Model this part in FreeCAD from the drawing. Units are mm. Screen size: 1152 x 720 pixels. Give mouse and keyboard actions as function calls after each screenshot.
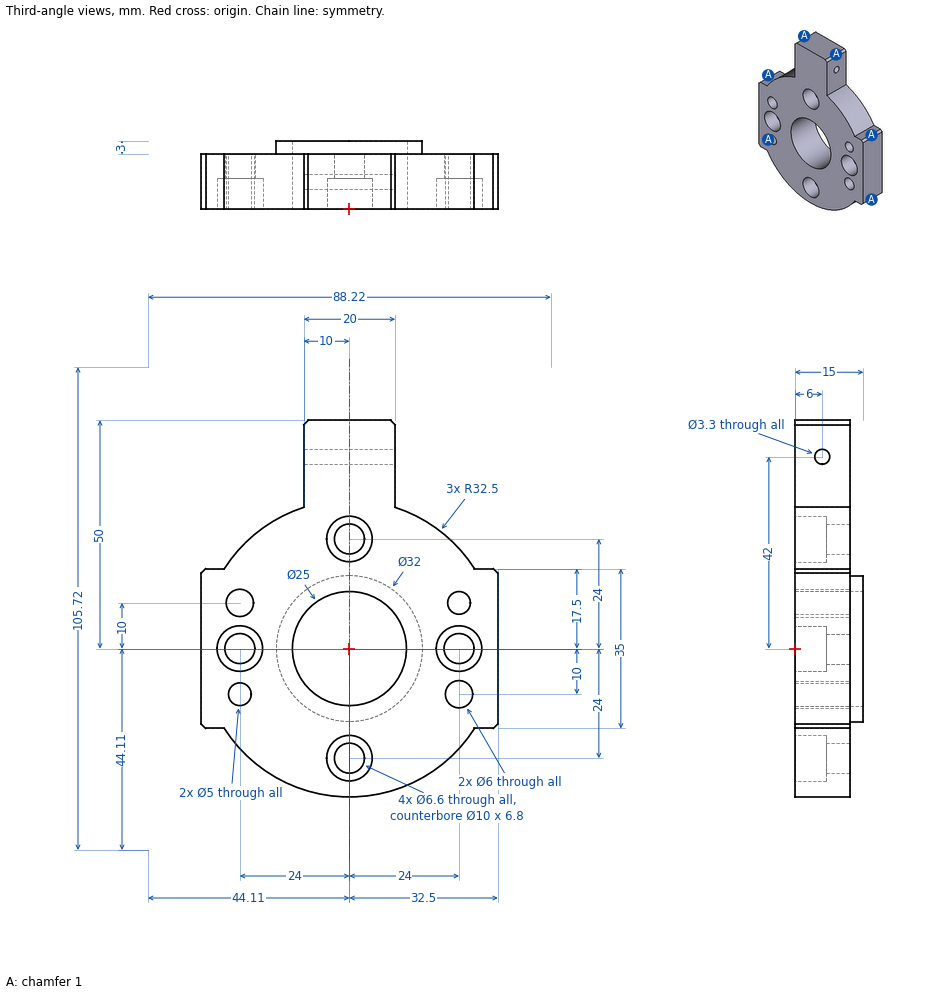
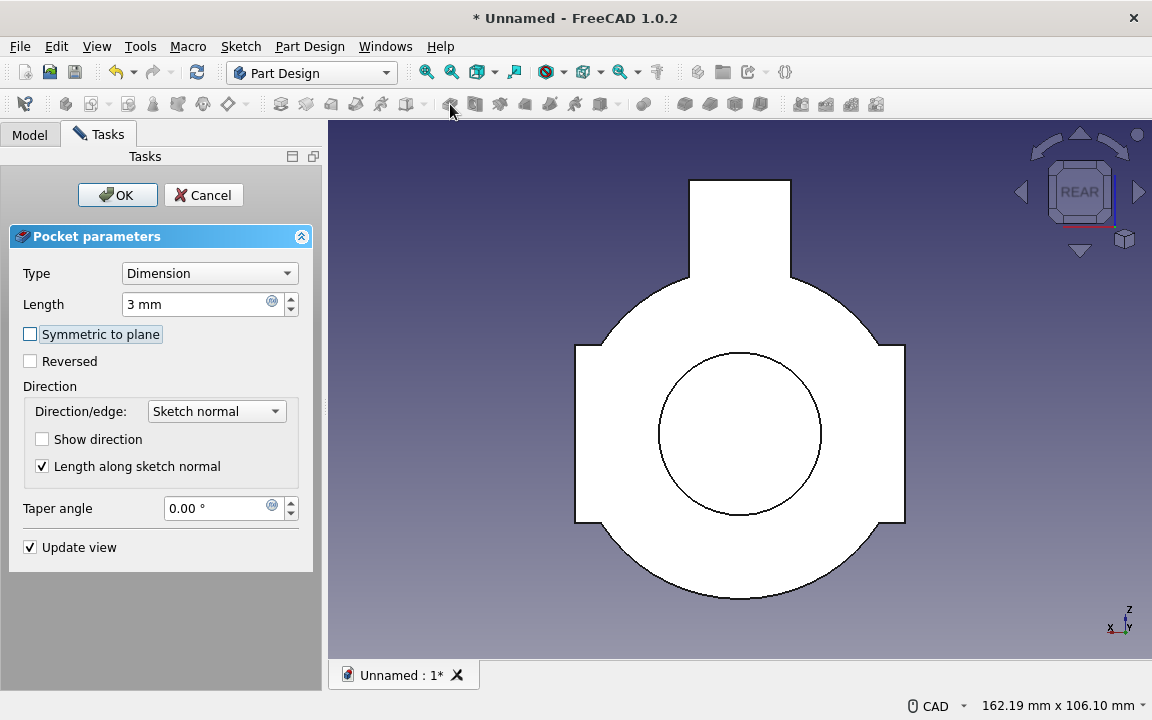
click(118, 195)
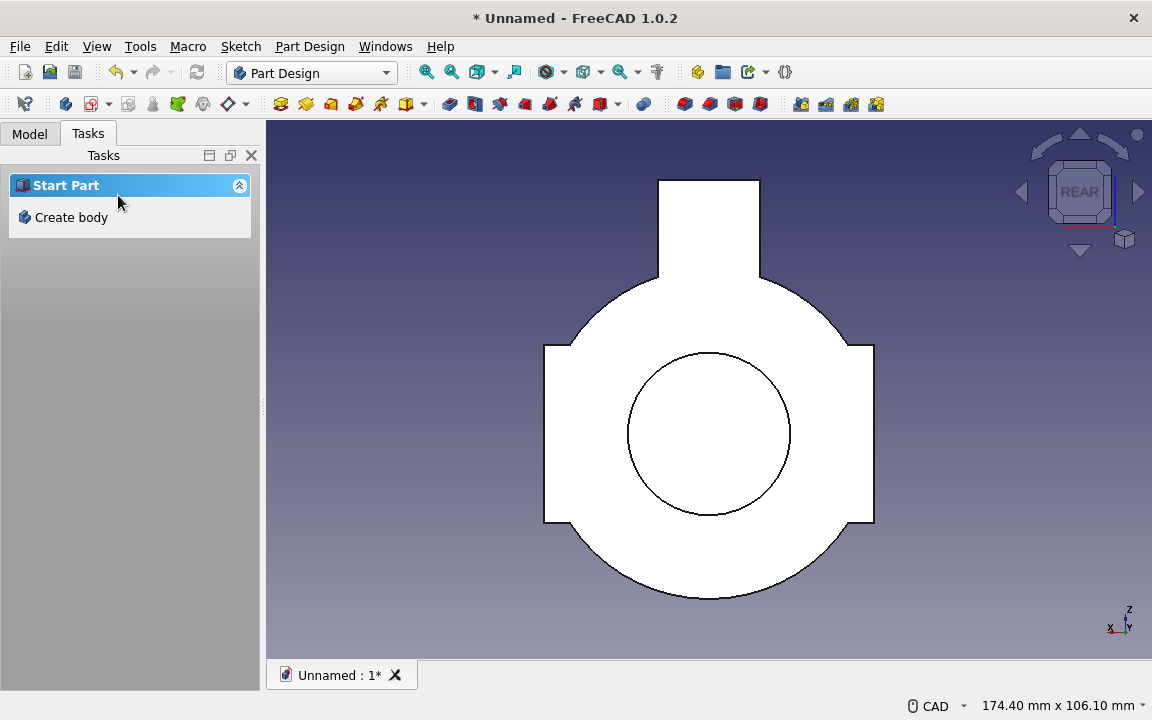
click(90, 104)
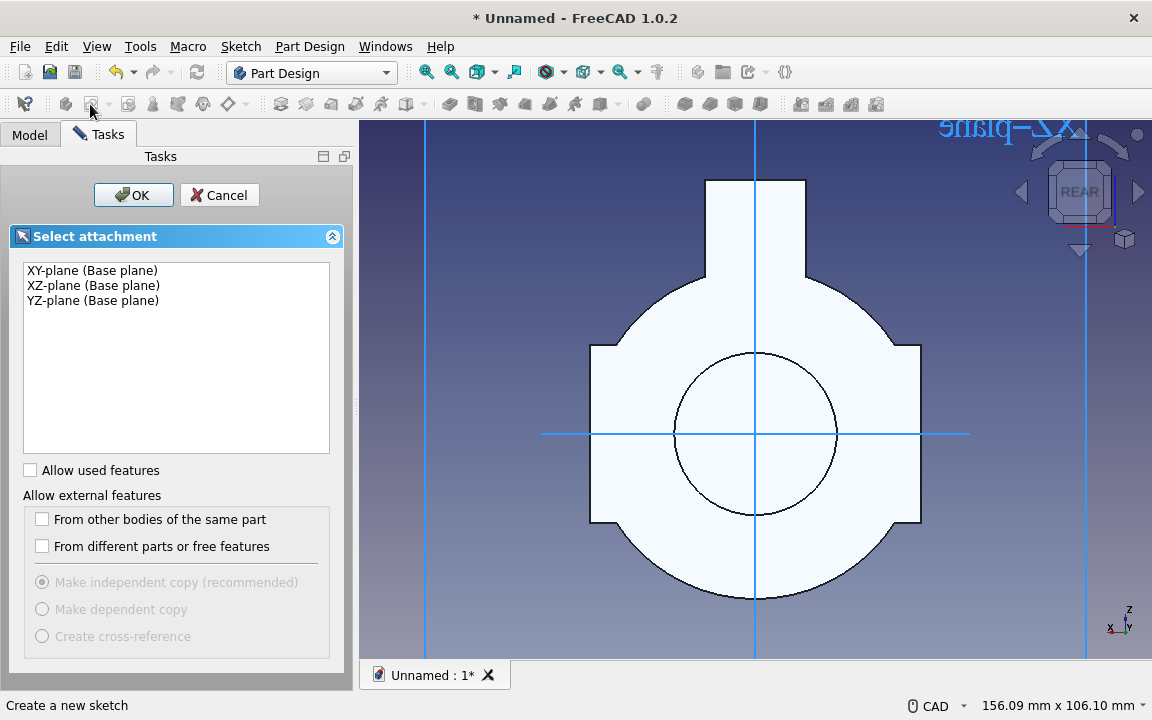
click(84, 286)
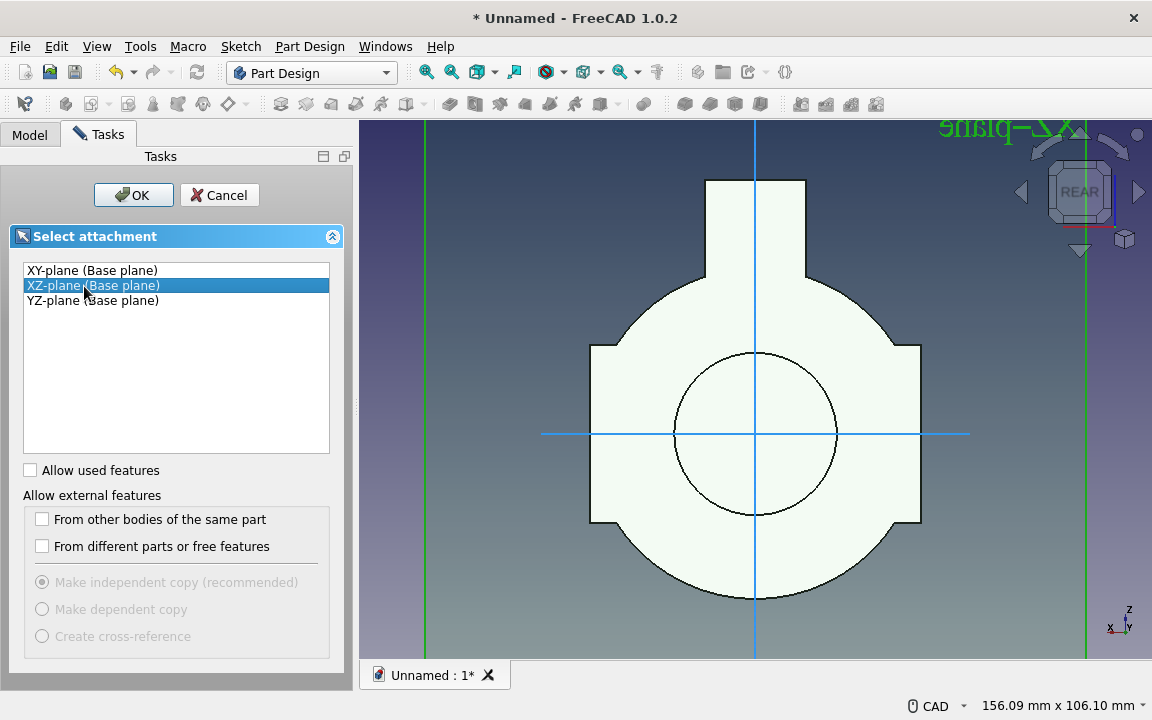
click(134, 195)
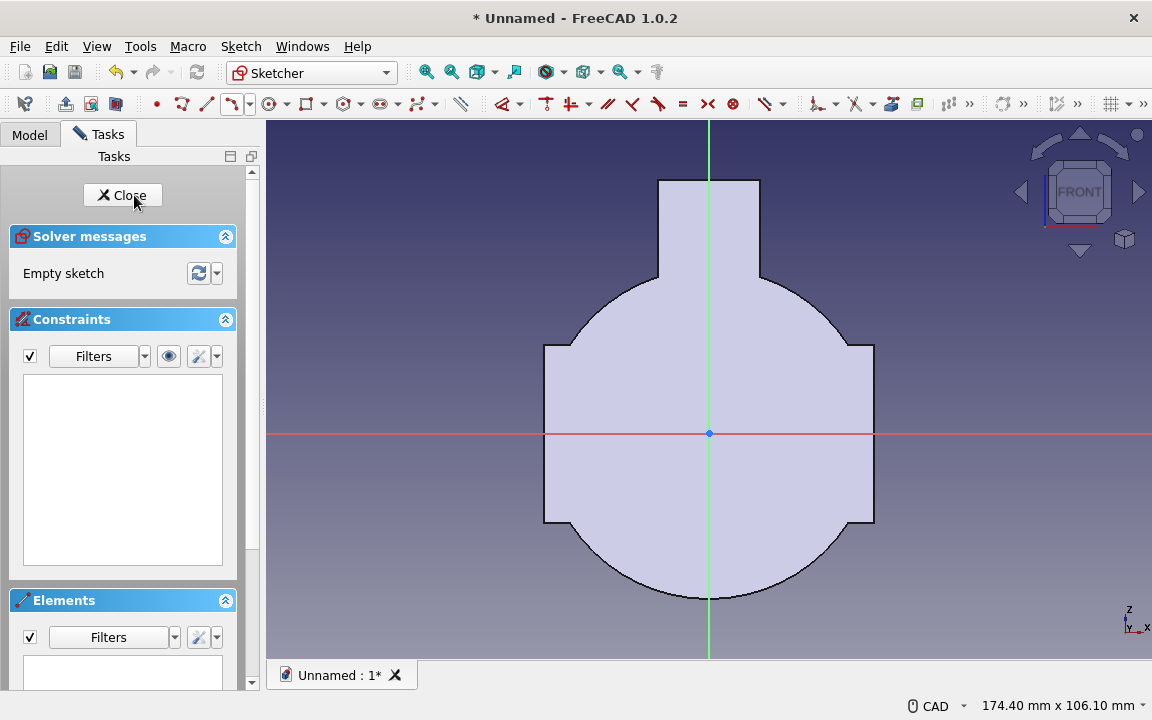
scroll(749, 460, up, 5)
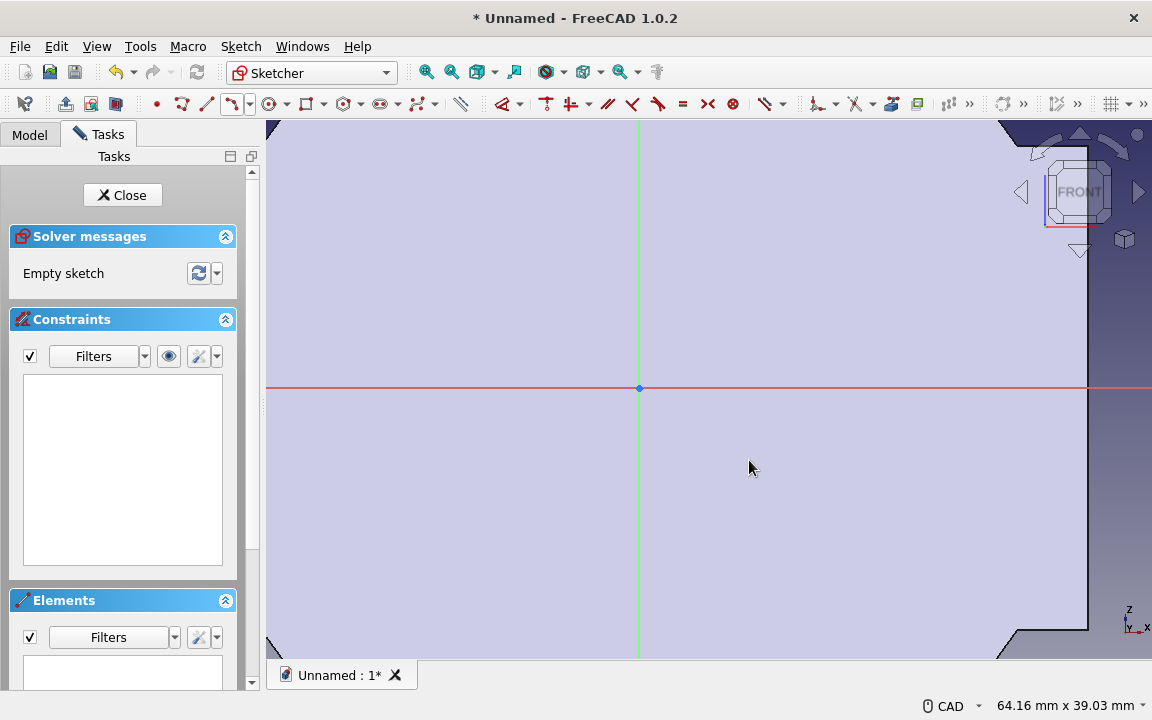
key(g)
key(c)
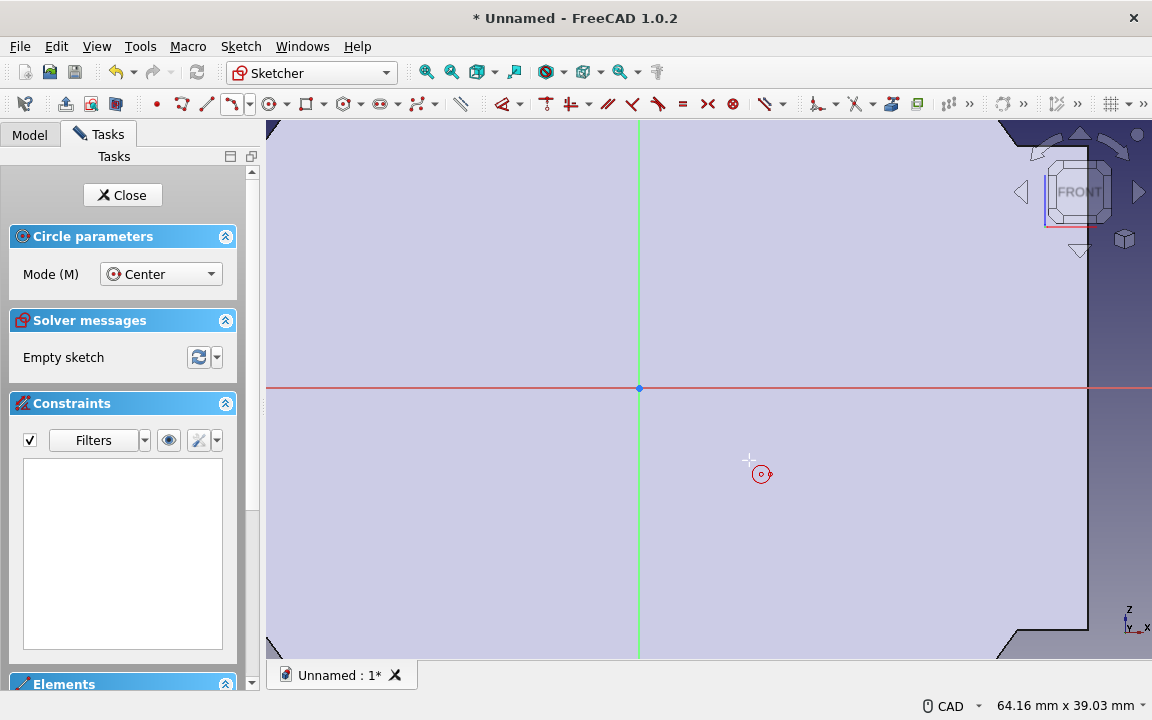
click(639, 388)
click(761, 266)
key(Escape)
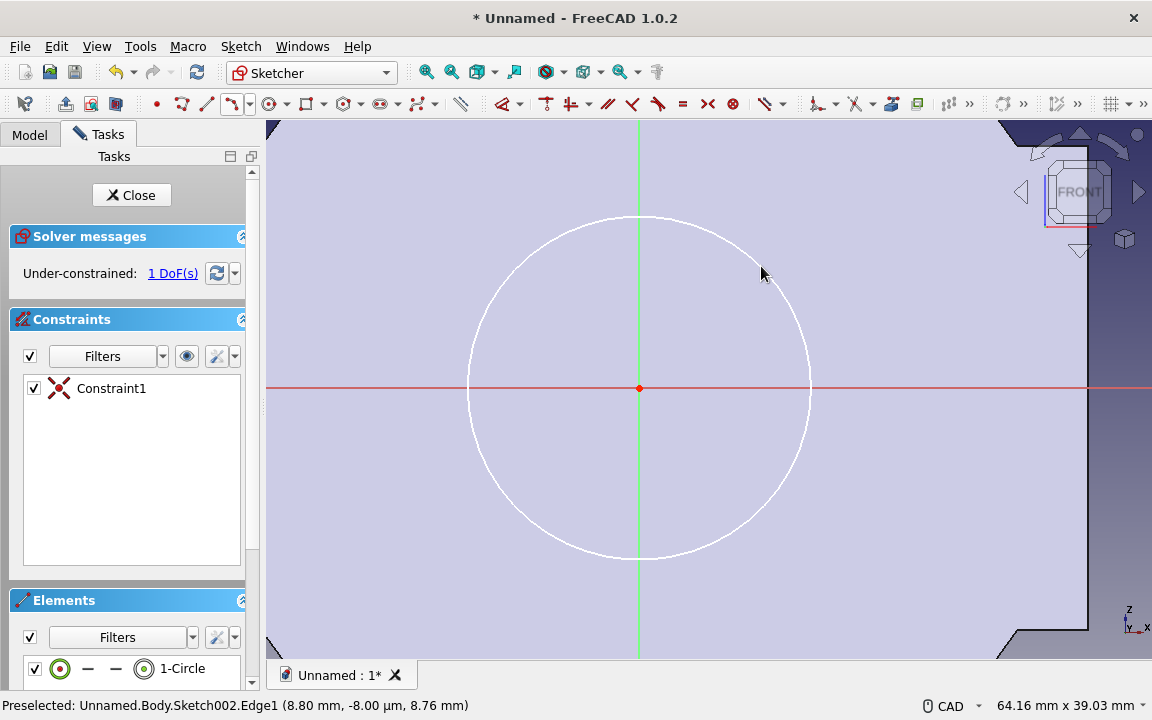
click(502, 104)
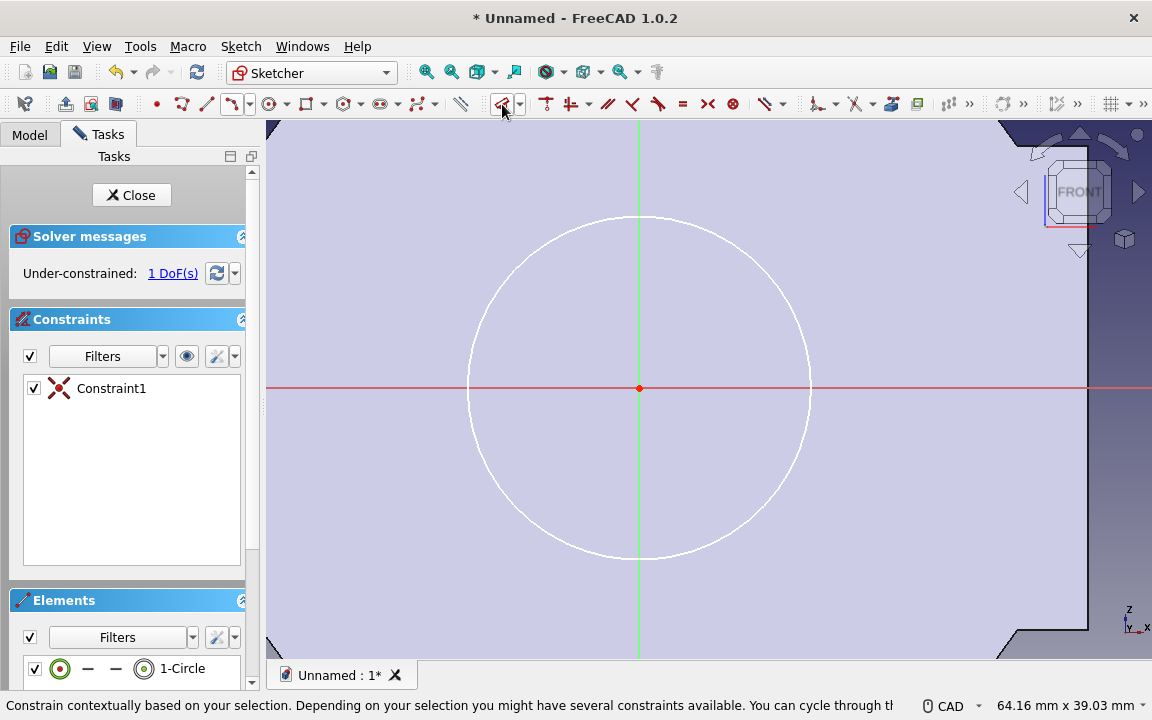
click(760, 266)
click(782, 243)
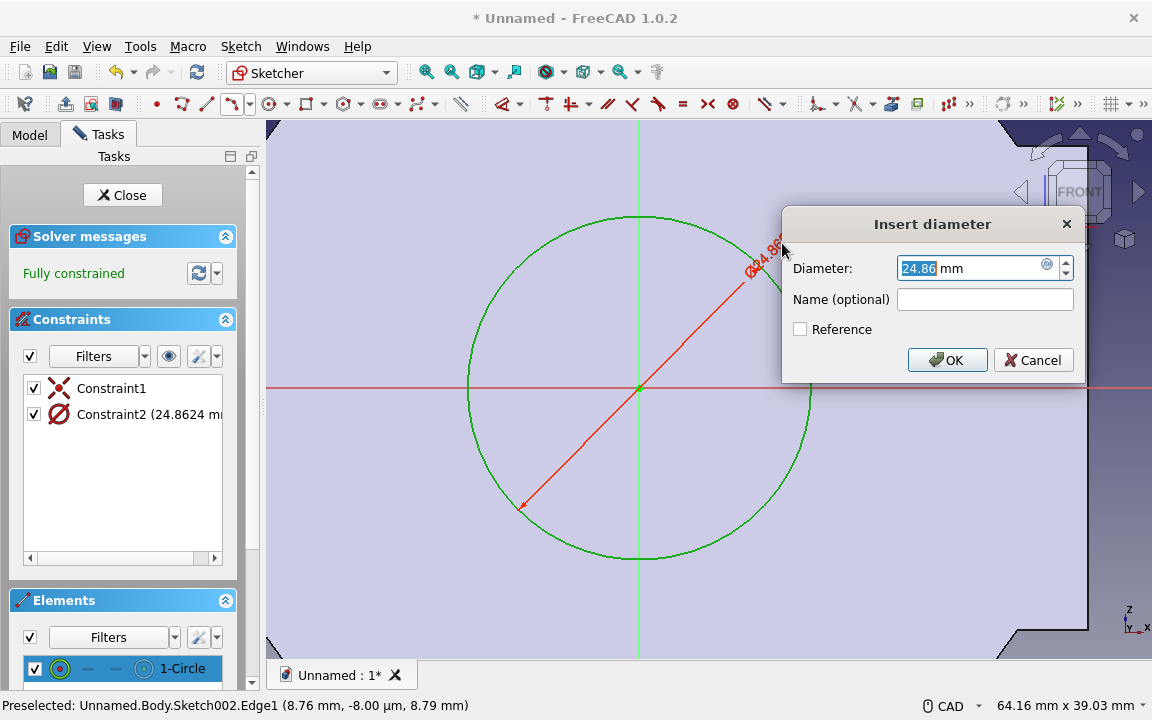
text(25)
key(Return)
key(Escape)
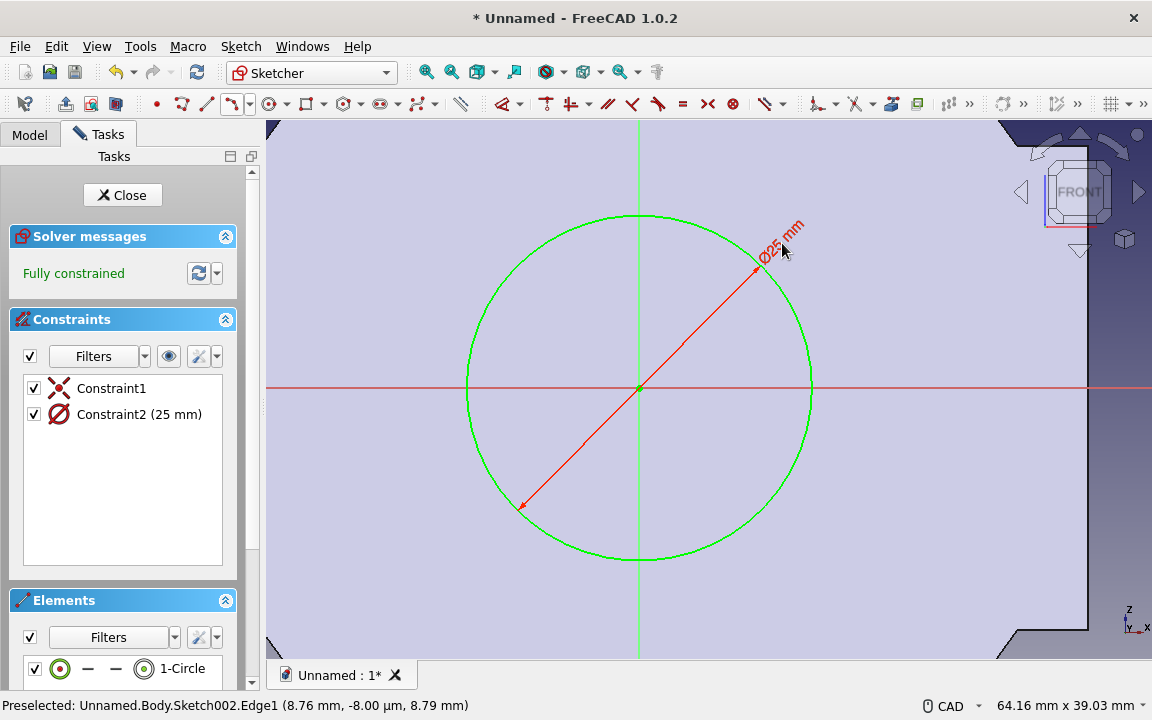
click(123, 195)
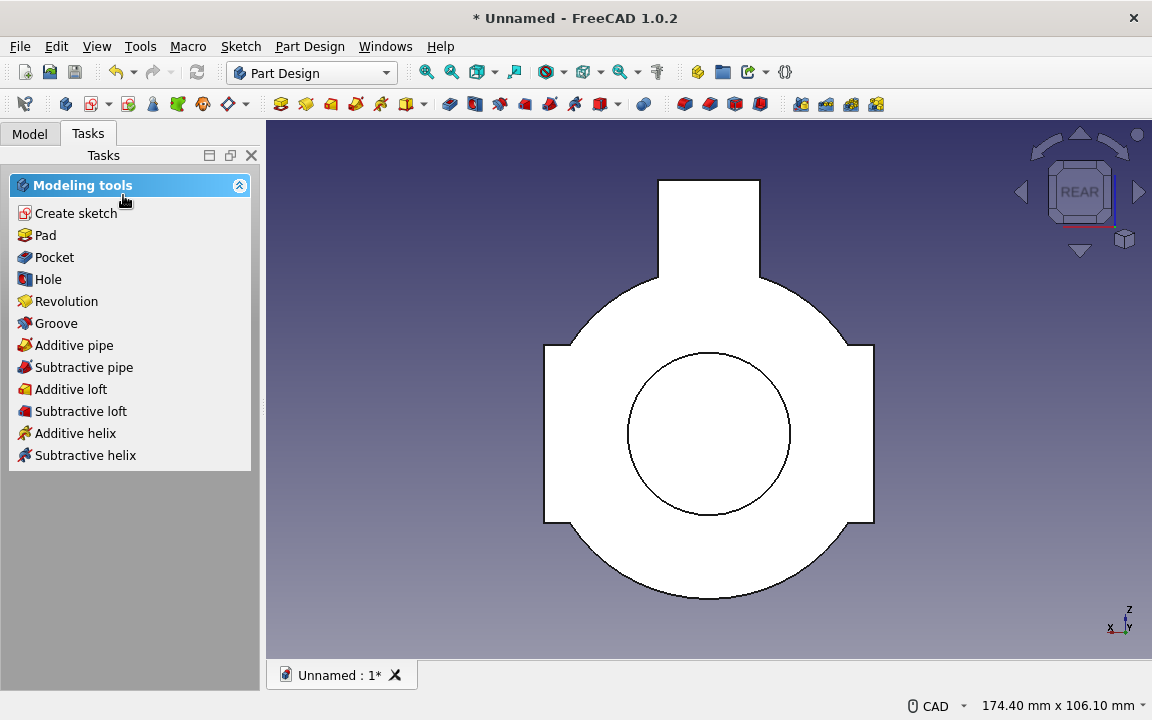
click(450, 104)